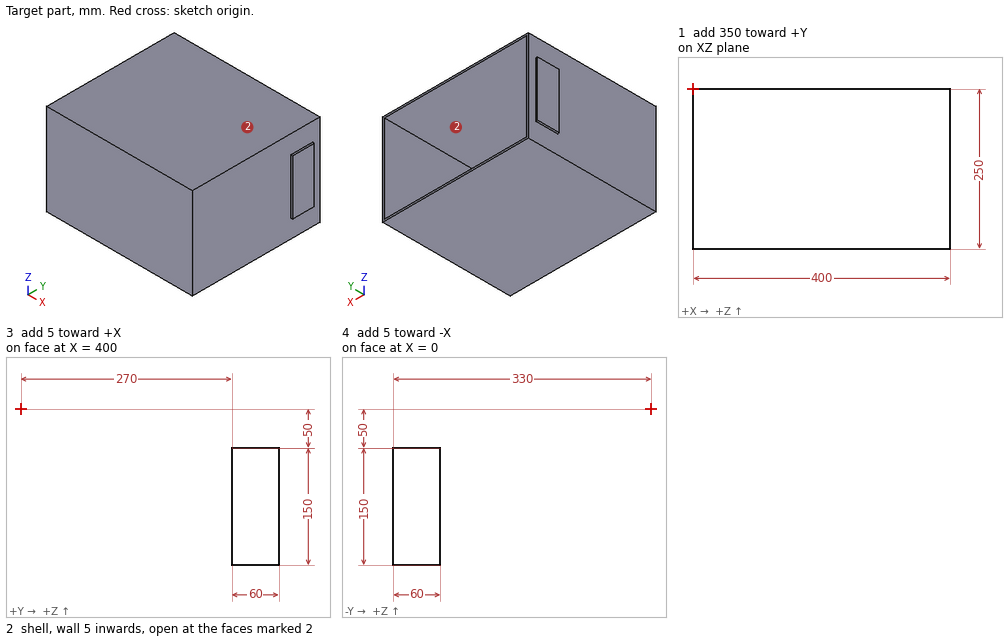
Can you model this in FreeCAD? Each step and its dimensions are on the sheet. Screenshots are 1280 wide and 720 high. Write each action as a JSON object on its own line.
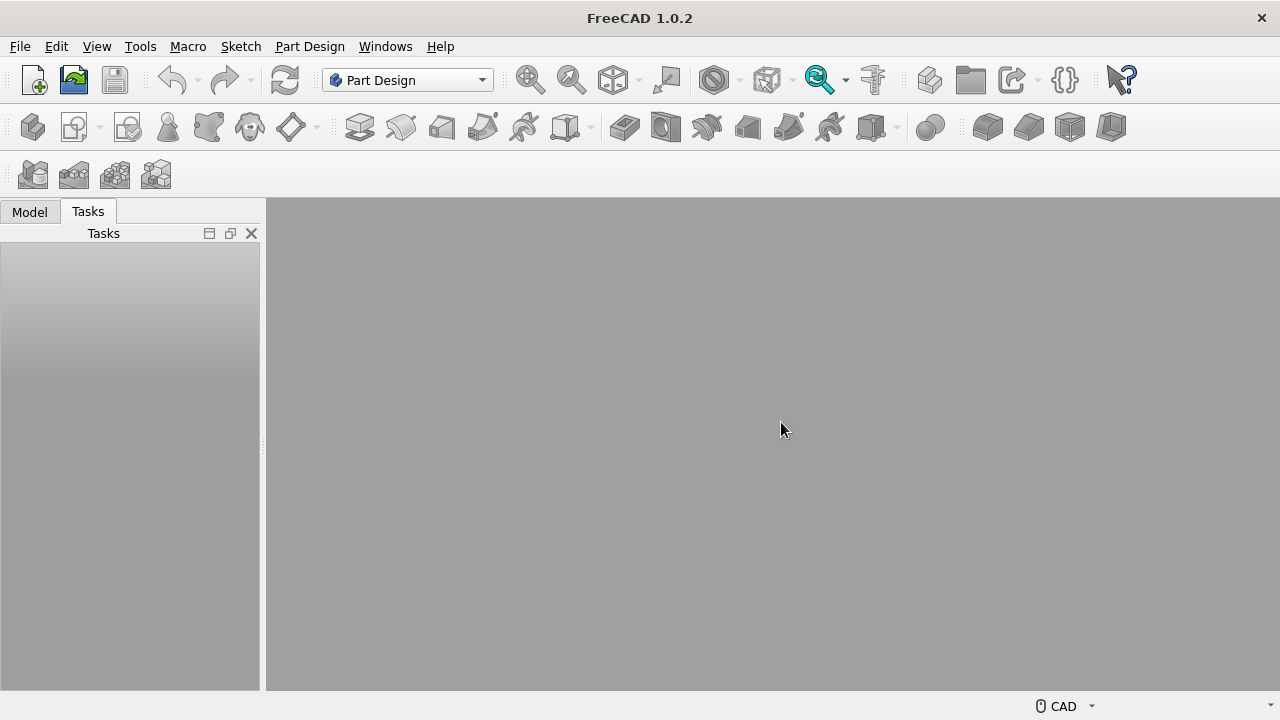
{"action": "key", "text": "ctrl+n"}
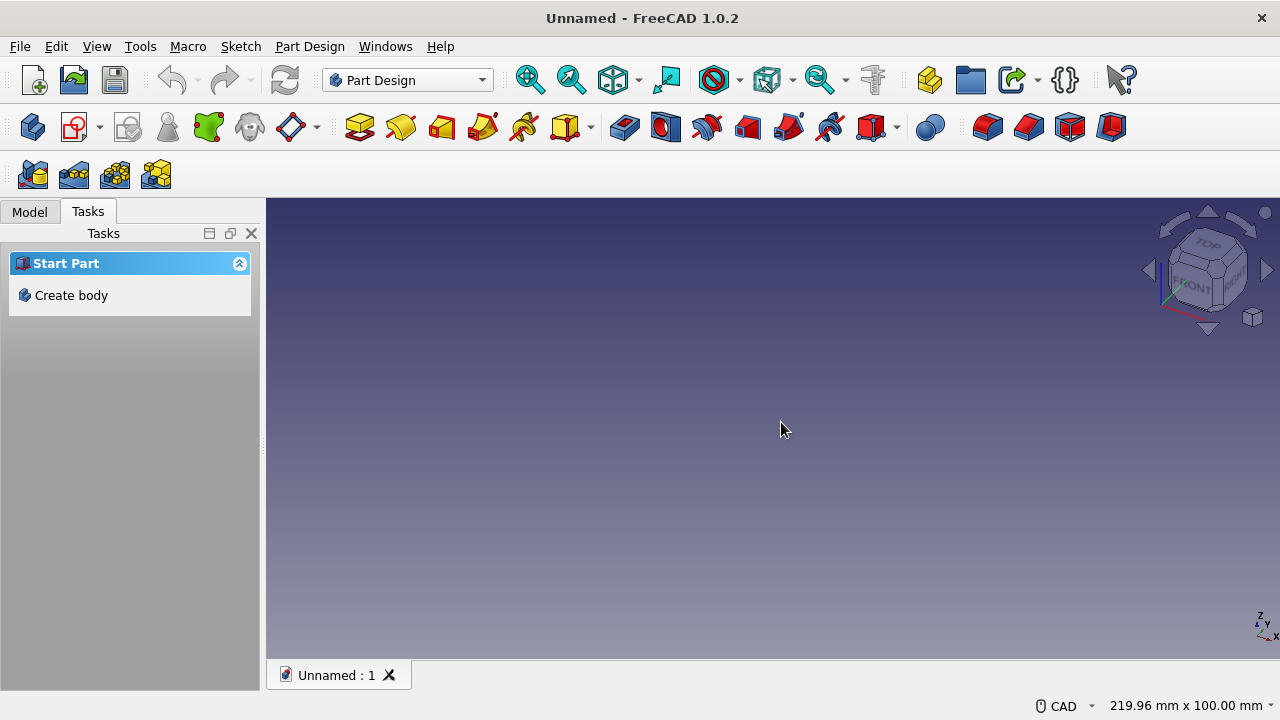
{"action": "left_click", "coordinate": [74, 128]}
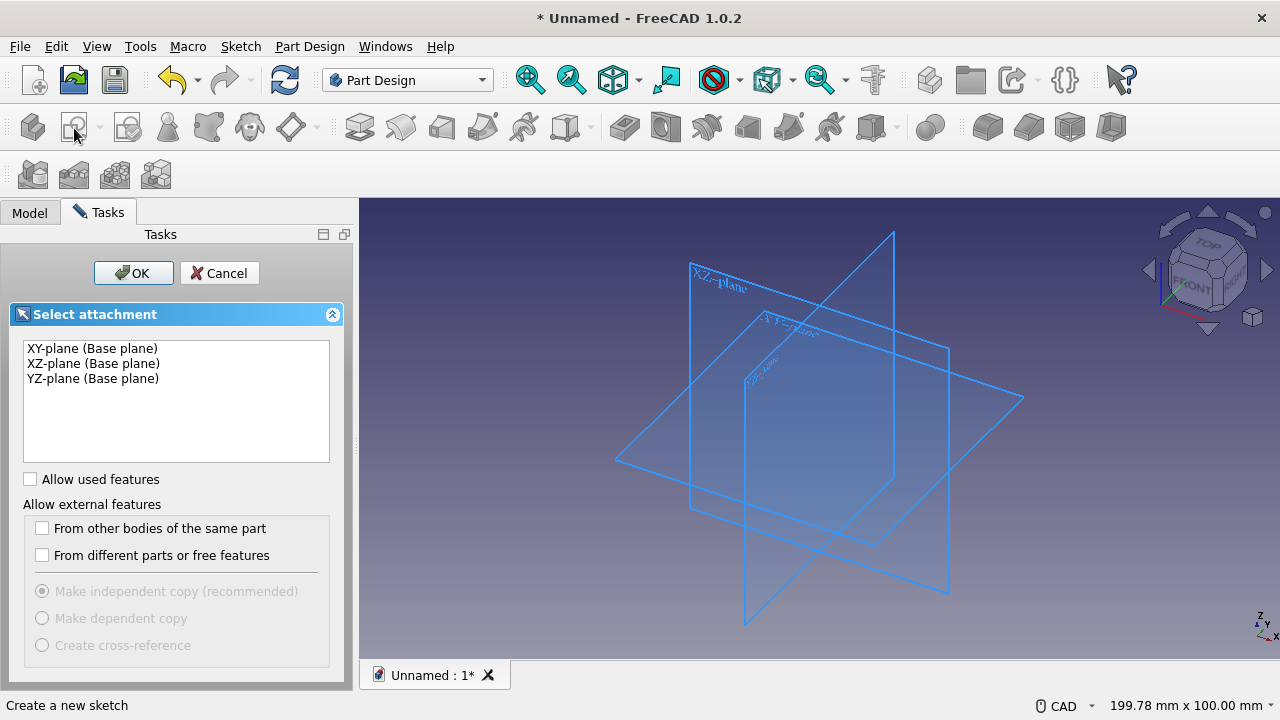
{"action": "left_click", "coordinate": [84, 364]}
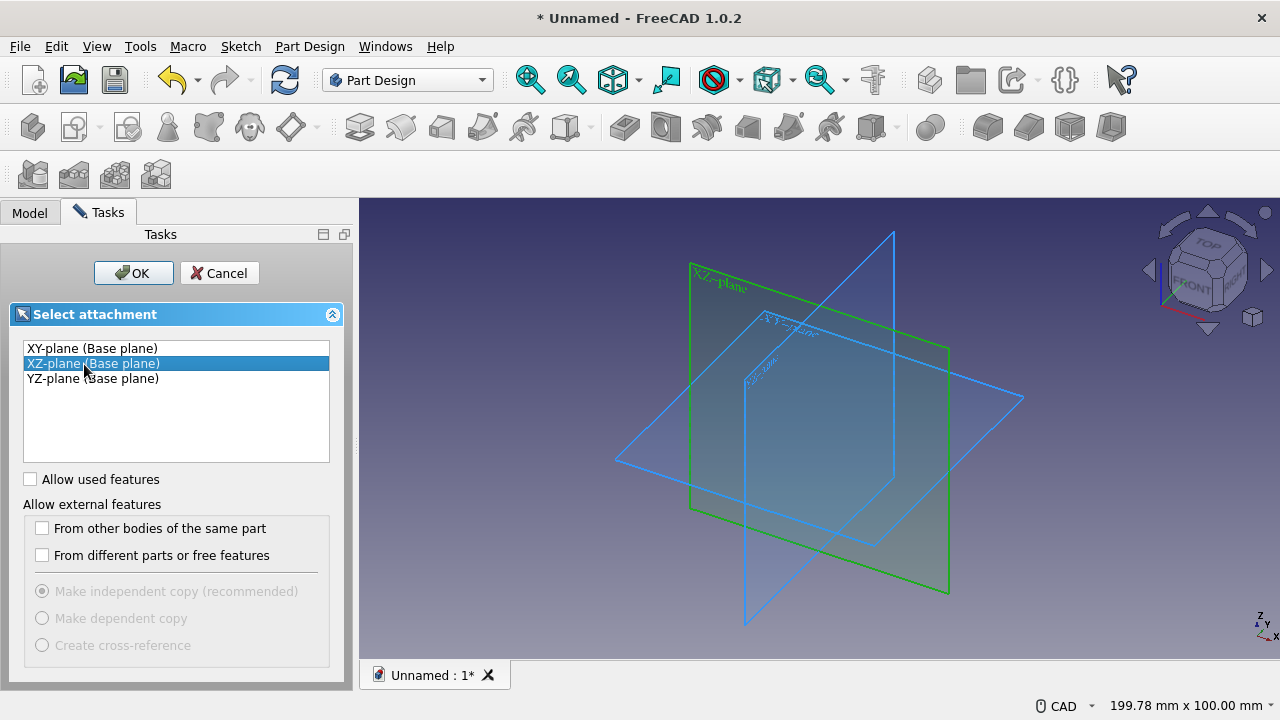
{"action": "left_click", "coordinate": [134, 273]}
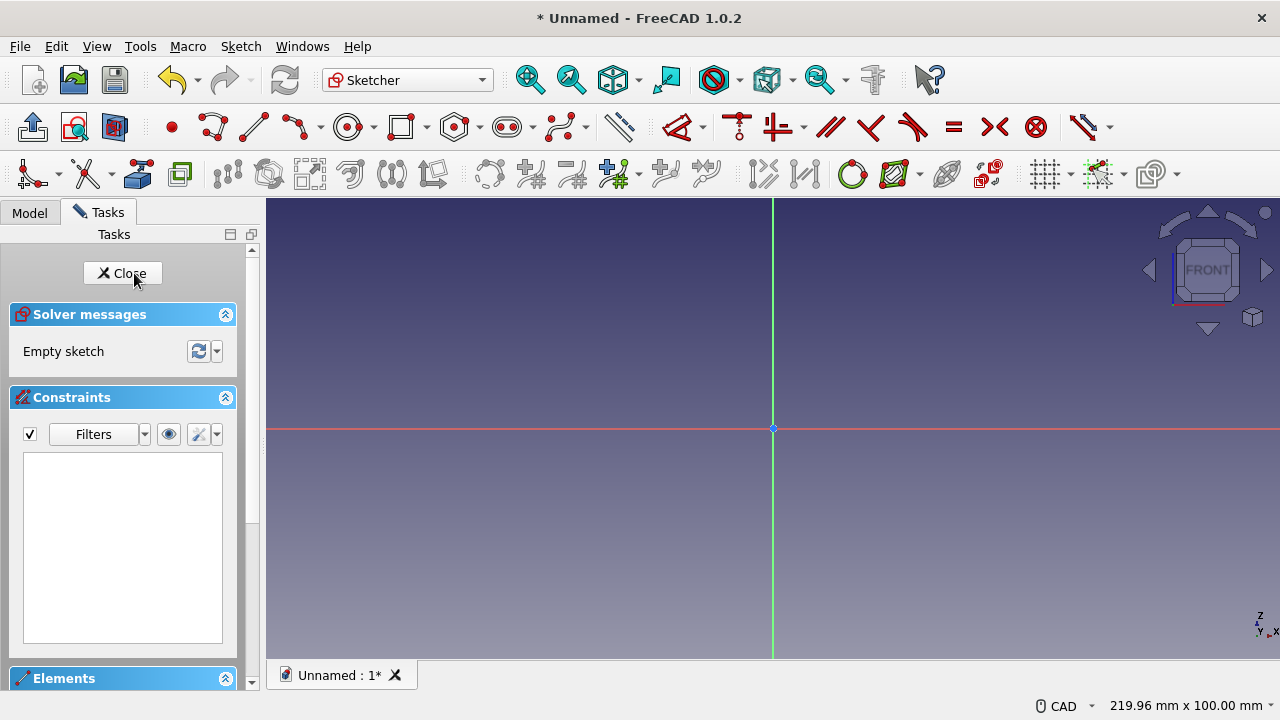
{"action": "scroll", "coordinate": [380, 240], "scroll_direction": "down", "scroll_amount": 7}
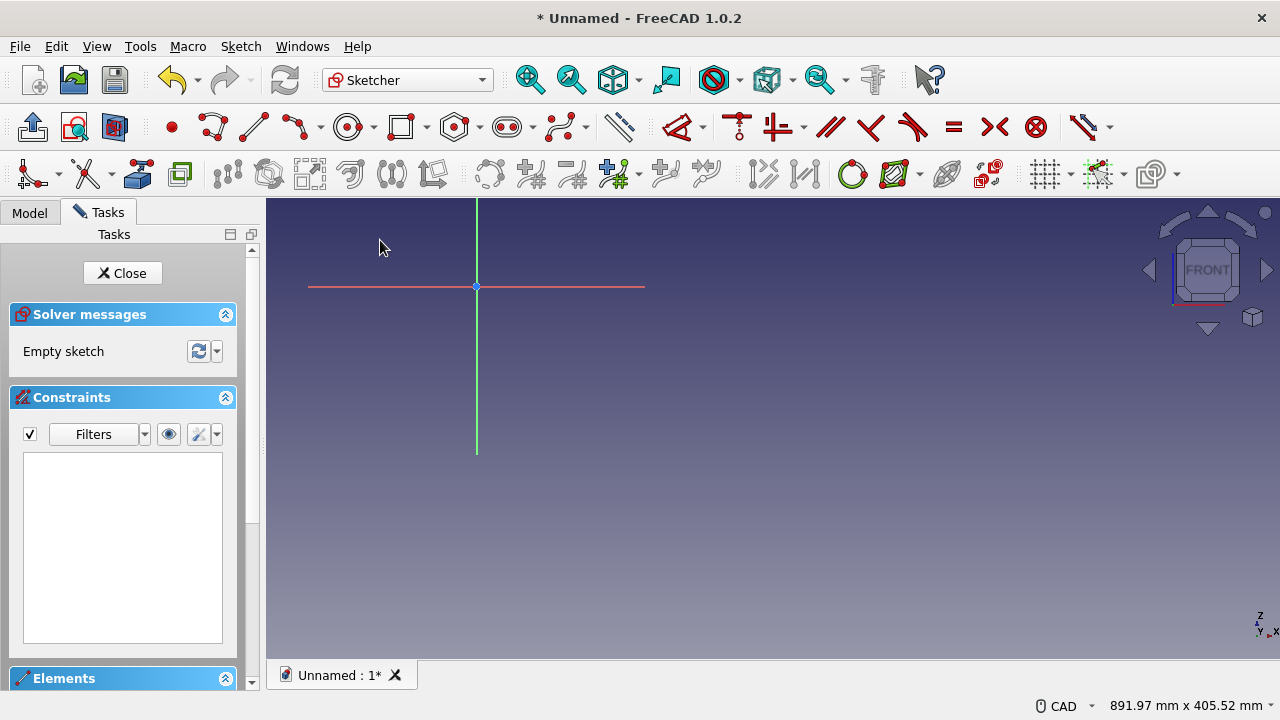
{"action": "key", "text": "g r"}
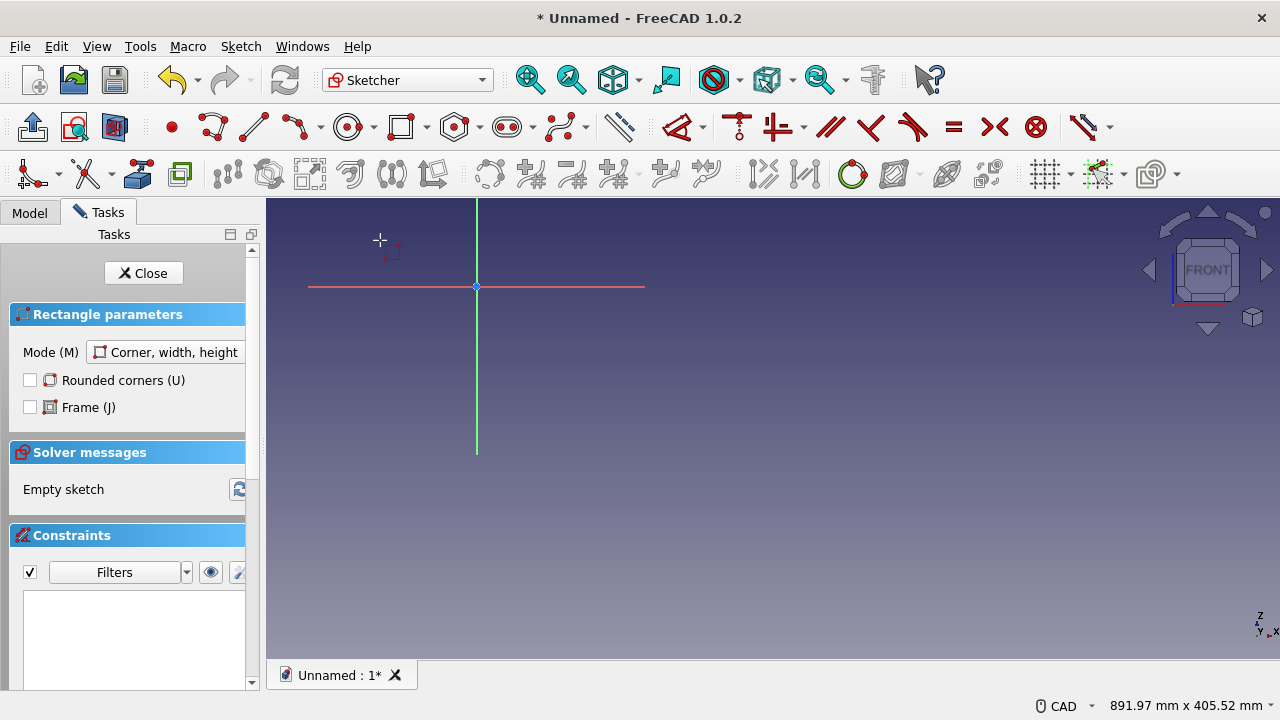
{"action": "left_click", "coordinate": [477, 287]}
{"action": "mouse_move", "coordinate": [932, 571]}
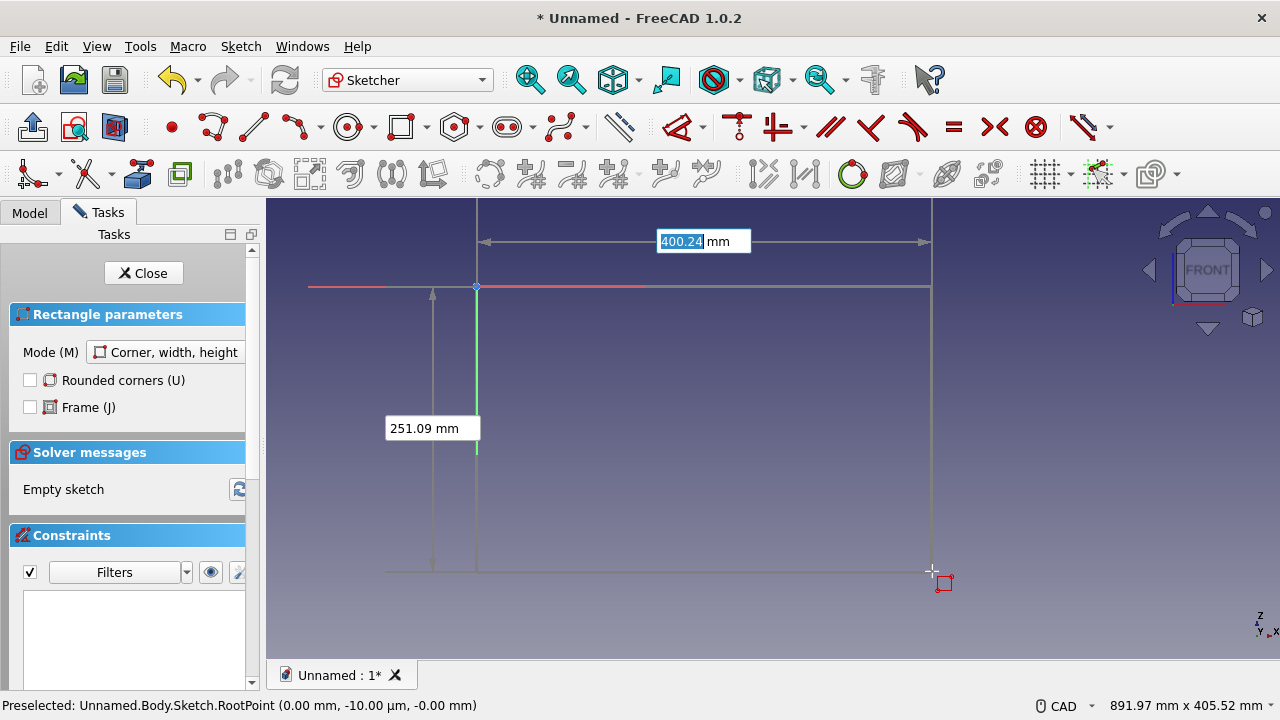
{"action": "type", "text": "400"}
{"action": "key", "text": "Tab"}
{"action": "type", "text": "250"}
{"action": "key", "text": "Return"}
{"action": "key", "text": "Escape"}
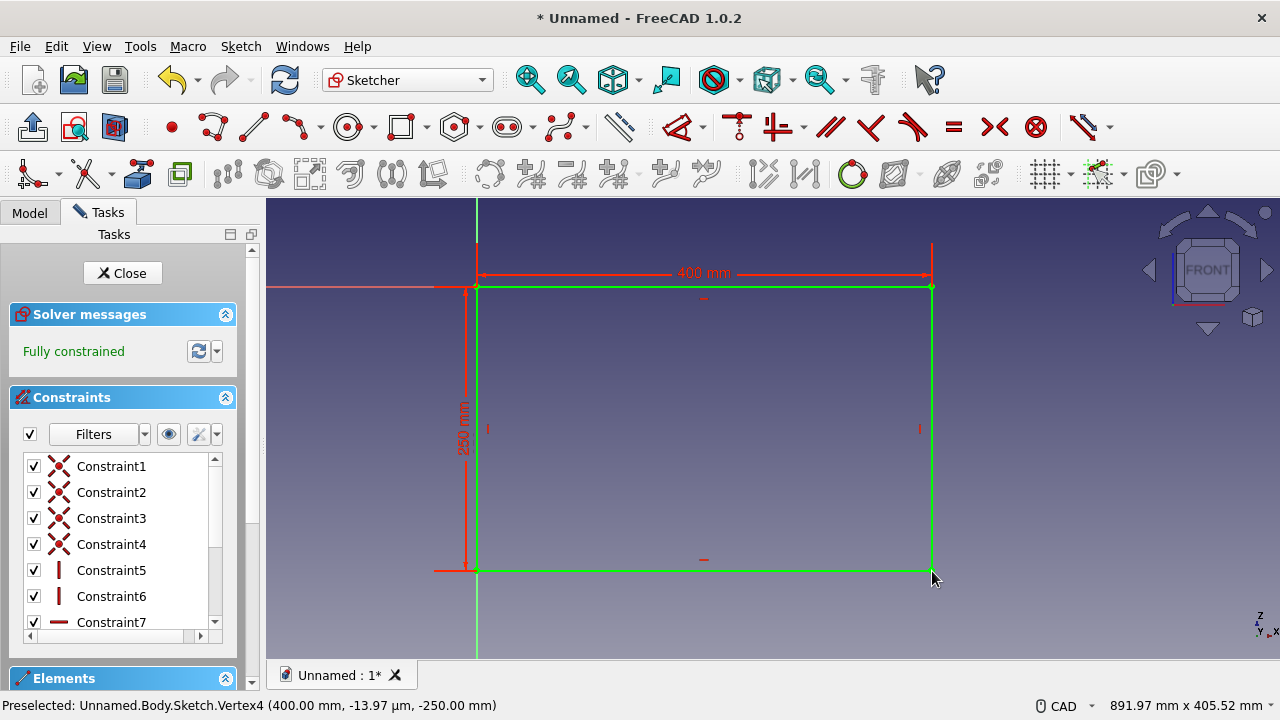
{"action": "left_click", "coordinate": [123, 273]}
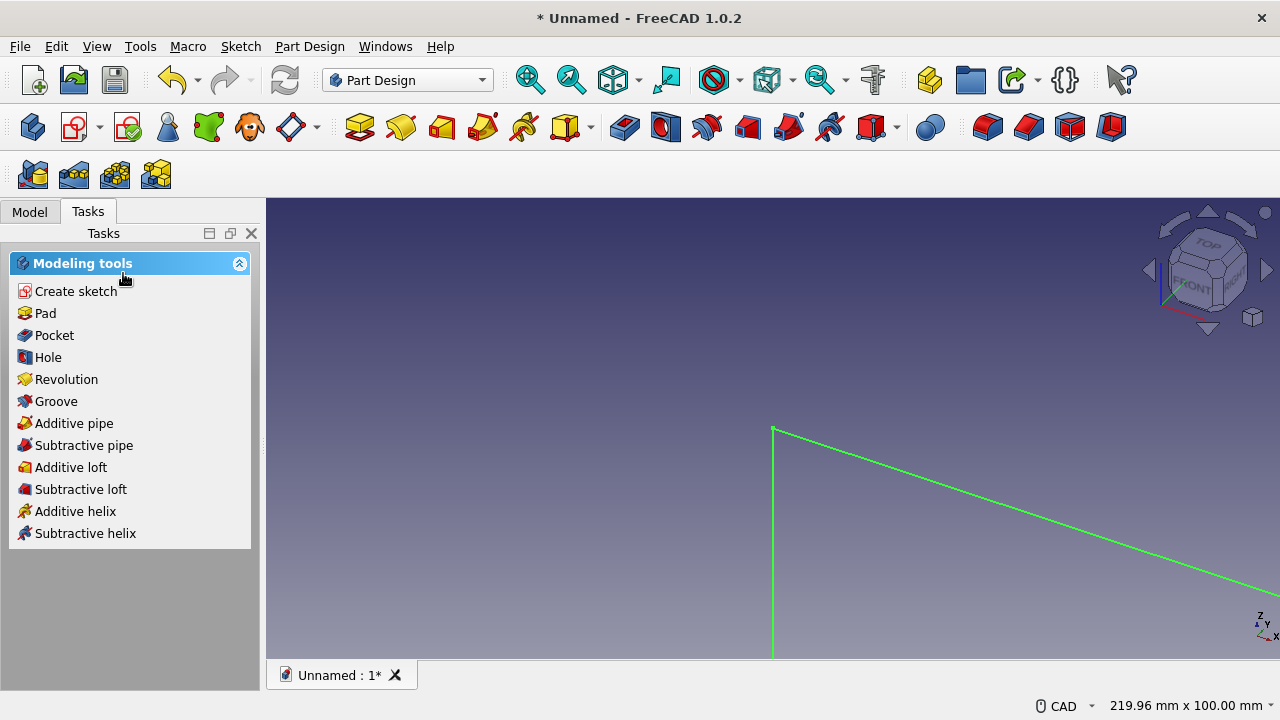
{"action": "left_click", "coordinate": [360, 128]}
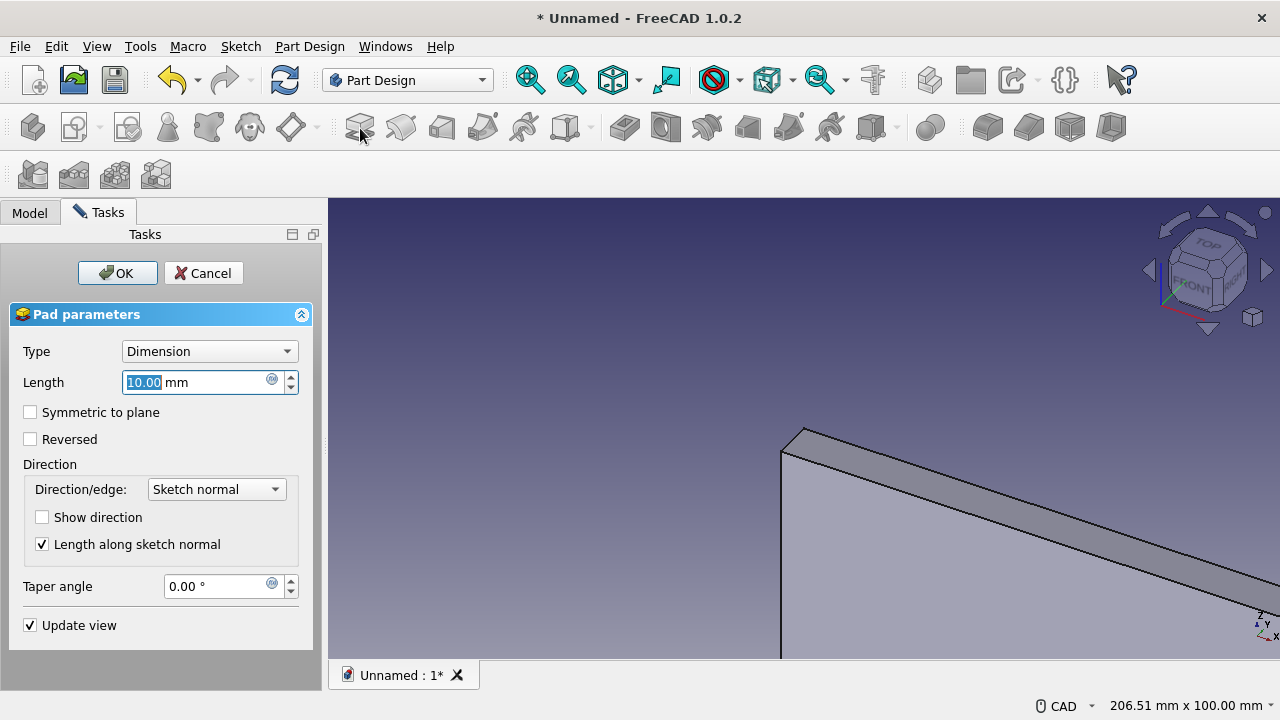
{"action": "type", "text": "350"}
{"action": "key", "text": "Tab"}